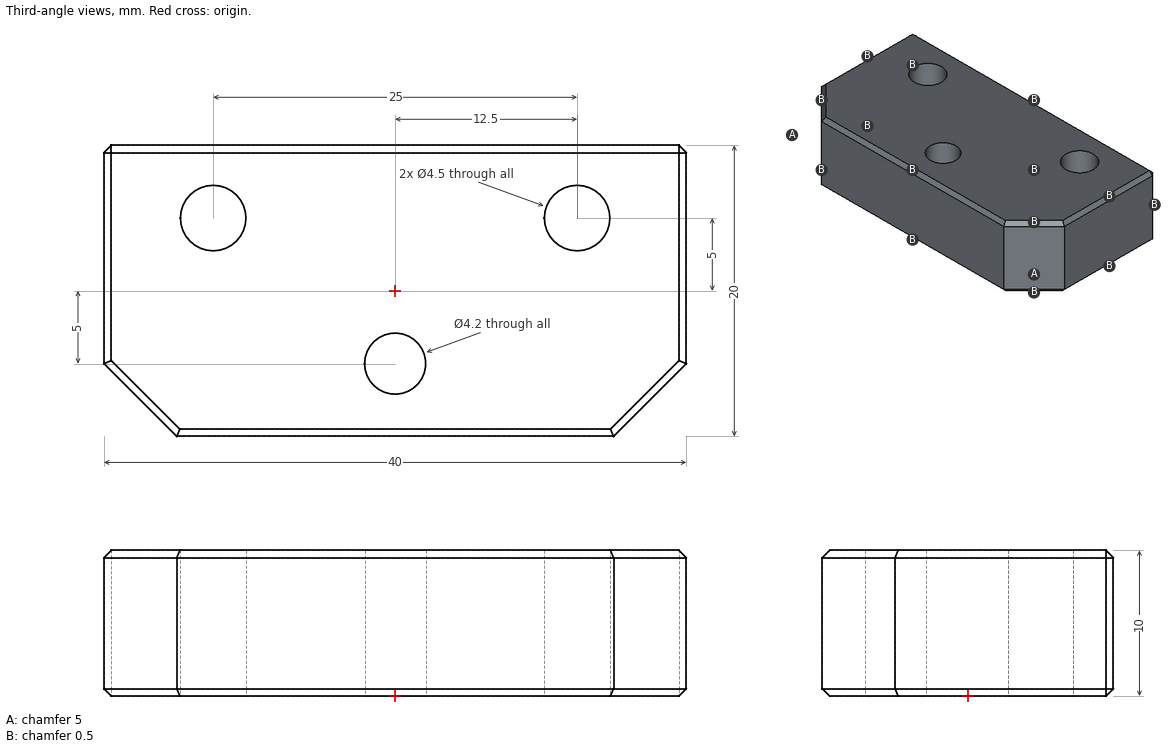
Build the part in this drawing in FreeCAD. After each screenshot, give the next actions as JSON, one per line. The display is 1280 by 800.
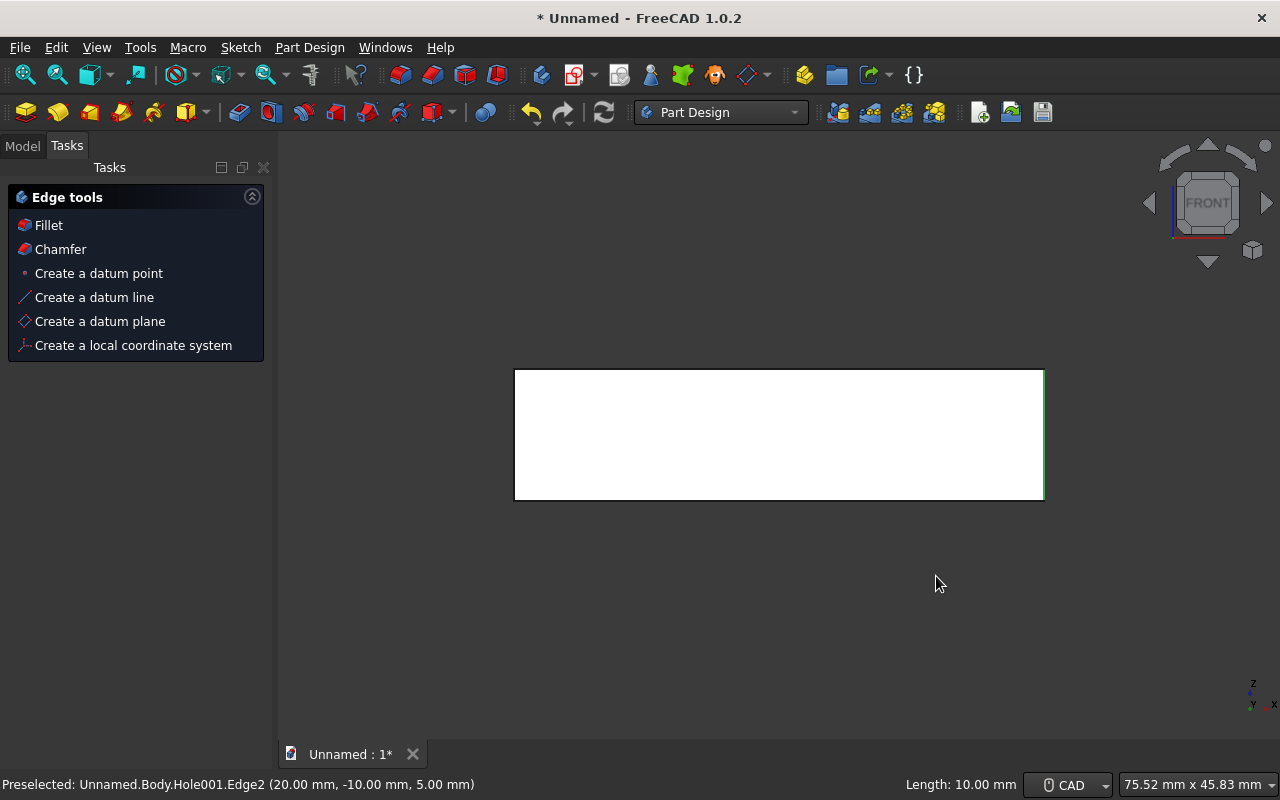
{"action": "left_click", "coordinate": [514, 434], "text": "ctrl"}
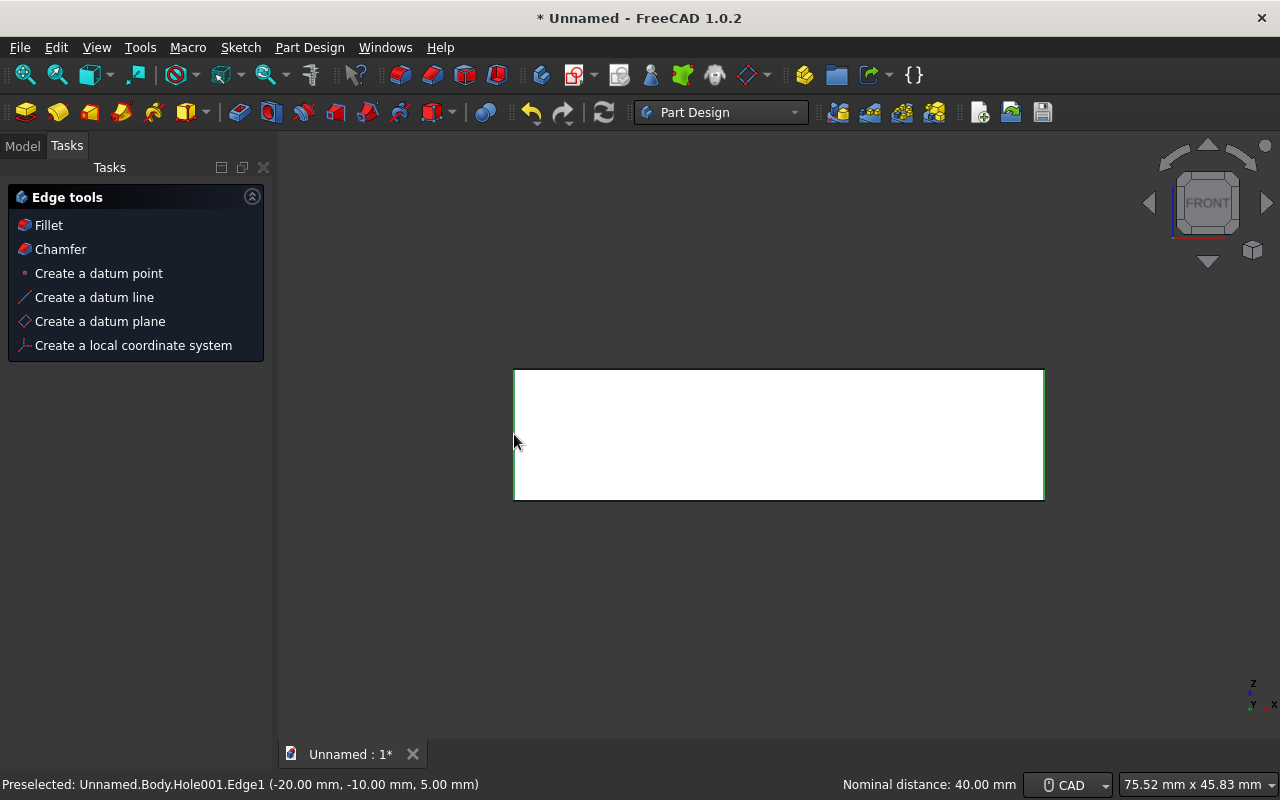
{"action": "left_click", "coordinate": [434, 76]}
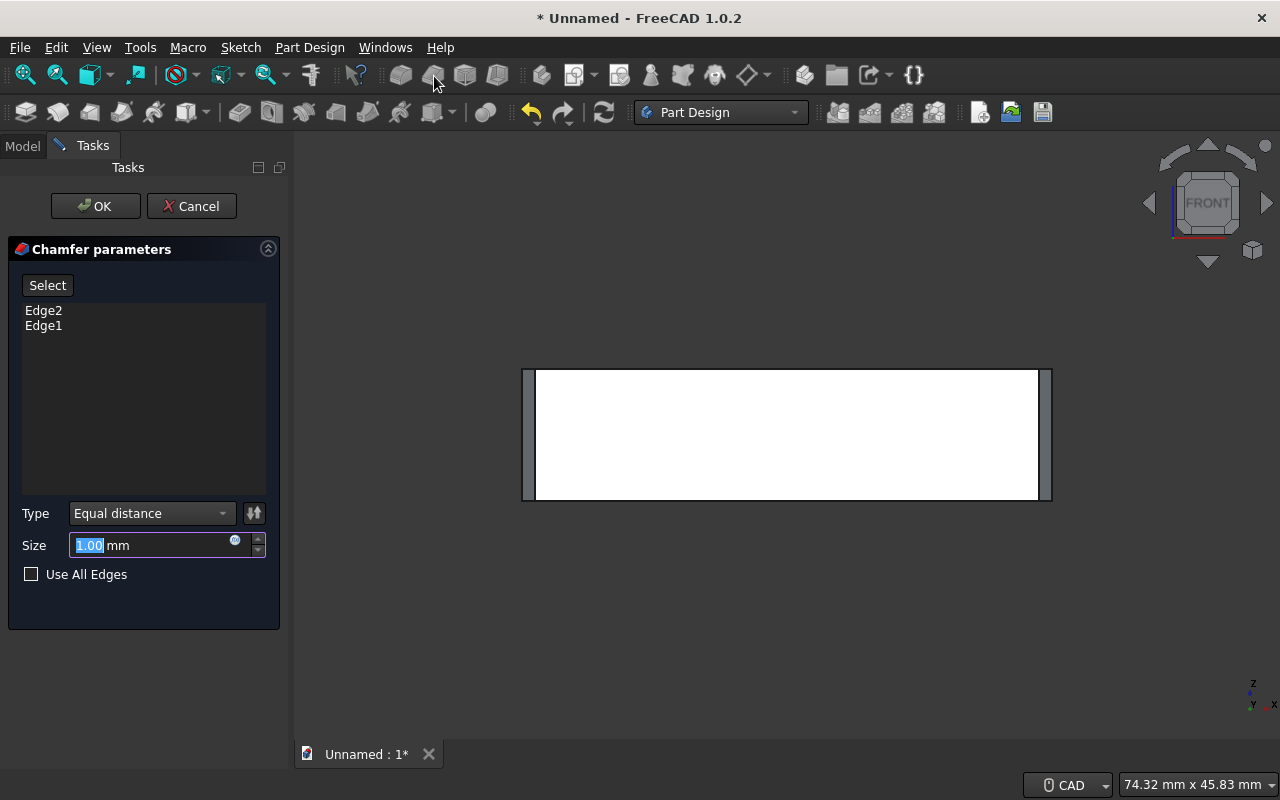
{"action": "type", "text": "5"}
{"action": "key", "text": "Tab"}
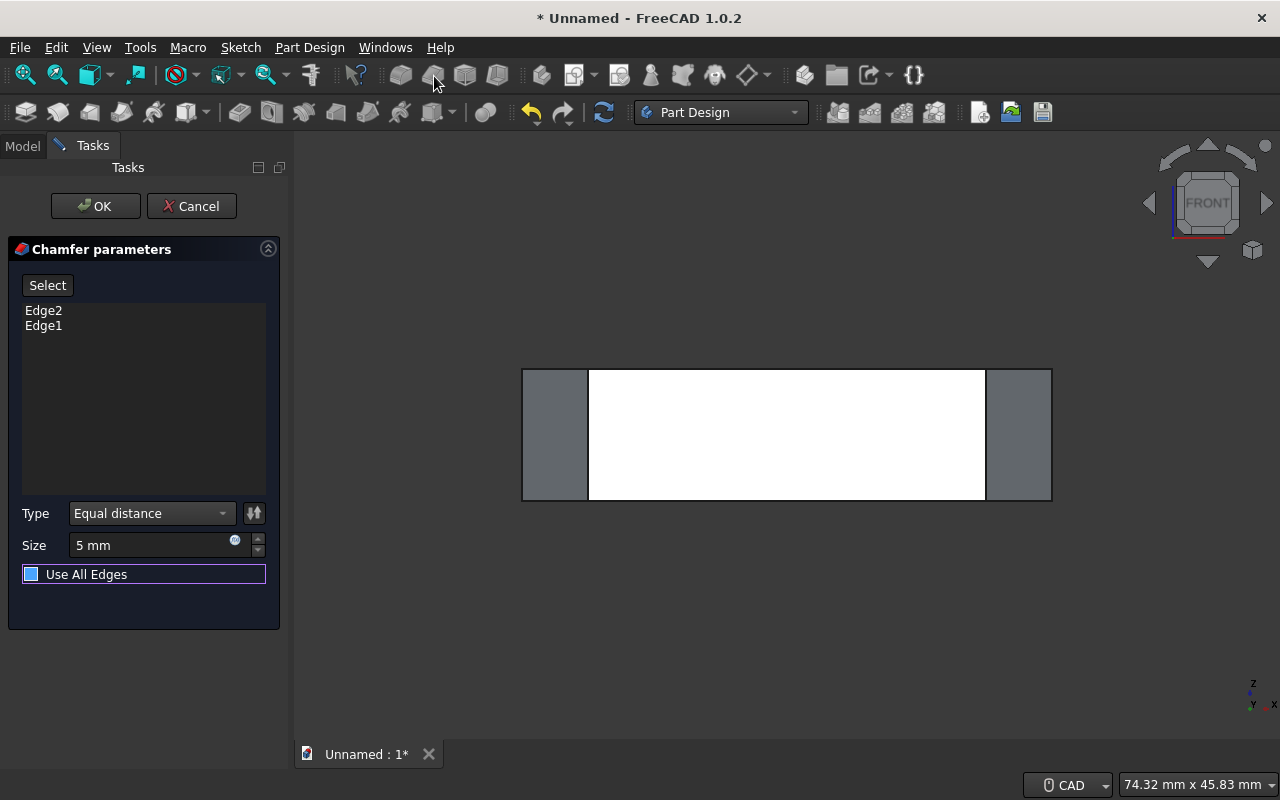
{"action": "left_click", "coordinate": [96, 206]}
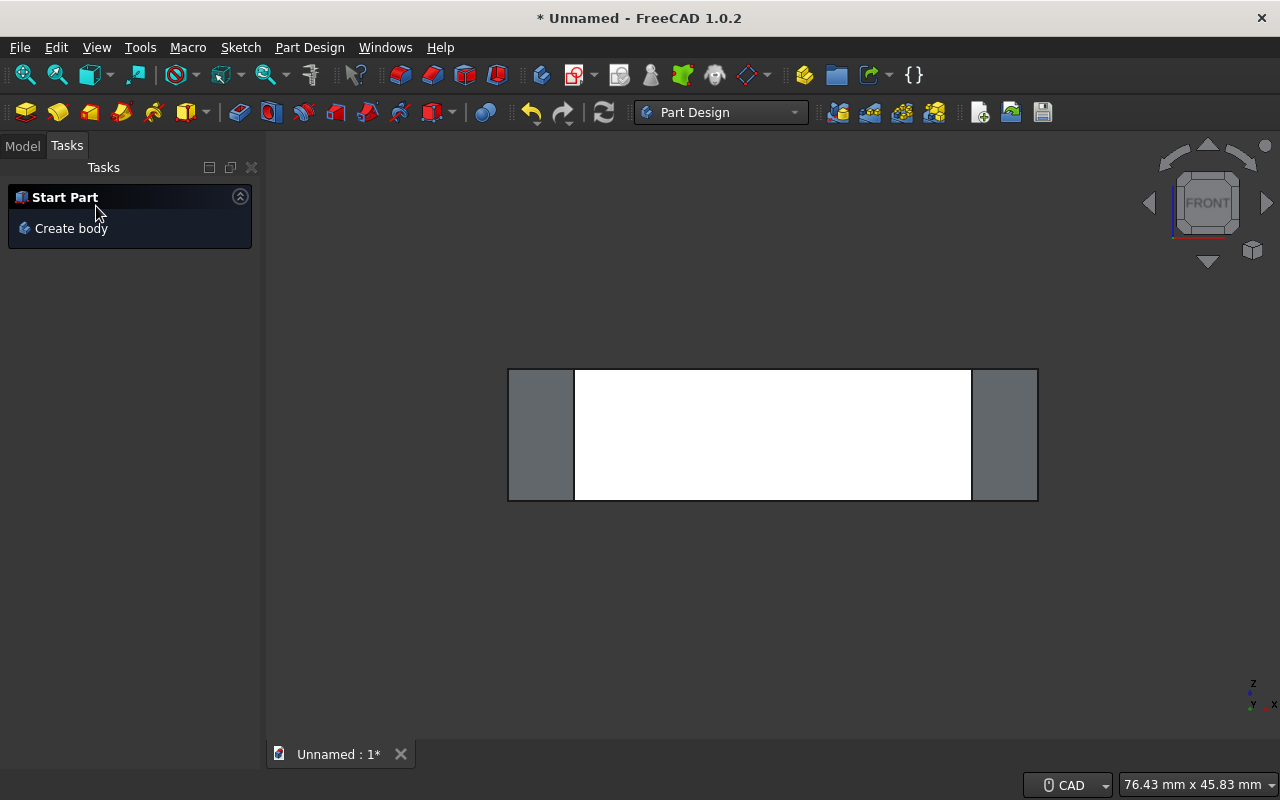
{"action": "left_click", "coordinate": [773, 500]}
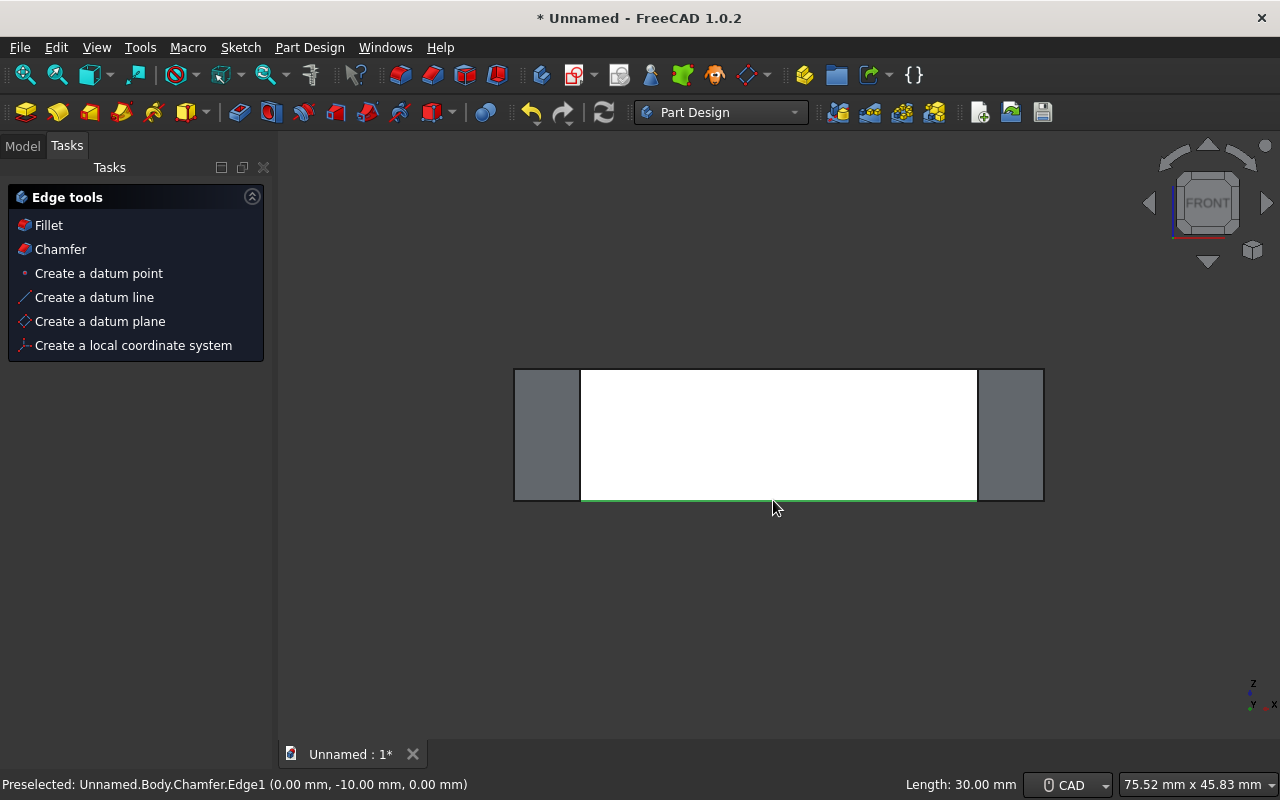
{"action": "left_click", "coordinate": [779, 368], "text": "ctrl"}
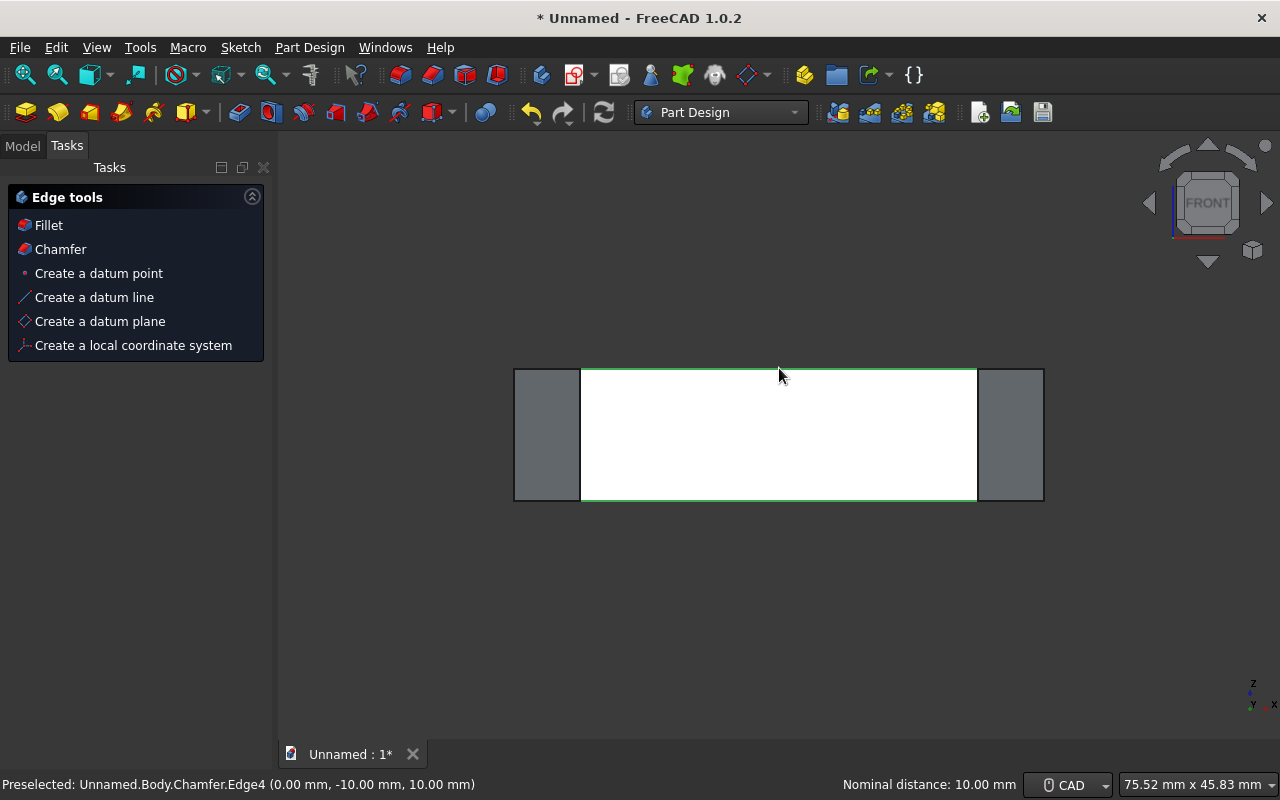
{"action": "left_click", "coordinate": [1011, 500], "text": "ctrl"}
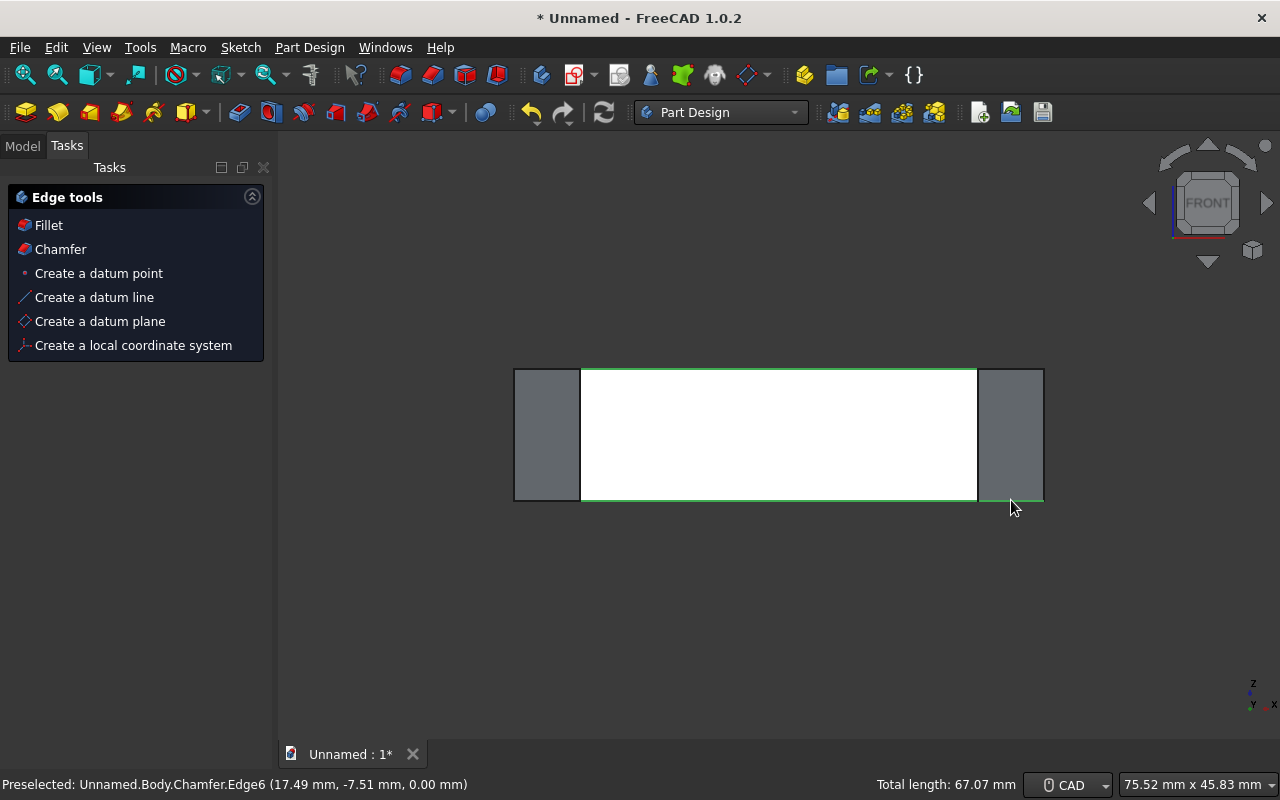
{"action": "left_click", "coordinate": [547, 500], "text": "ctrl"}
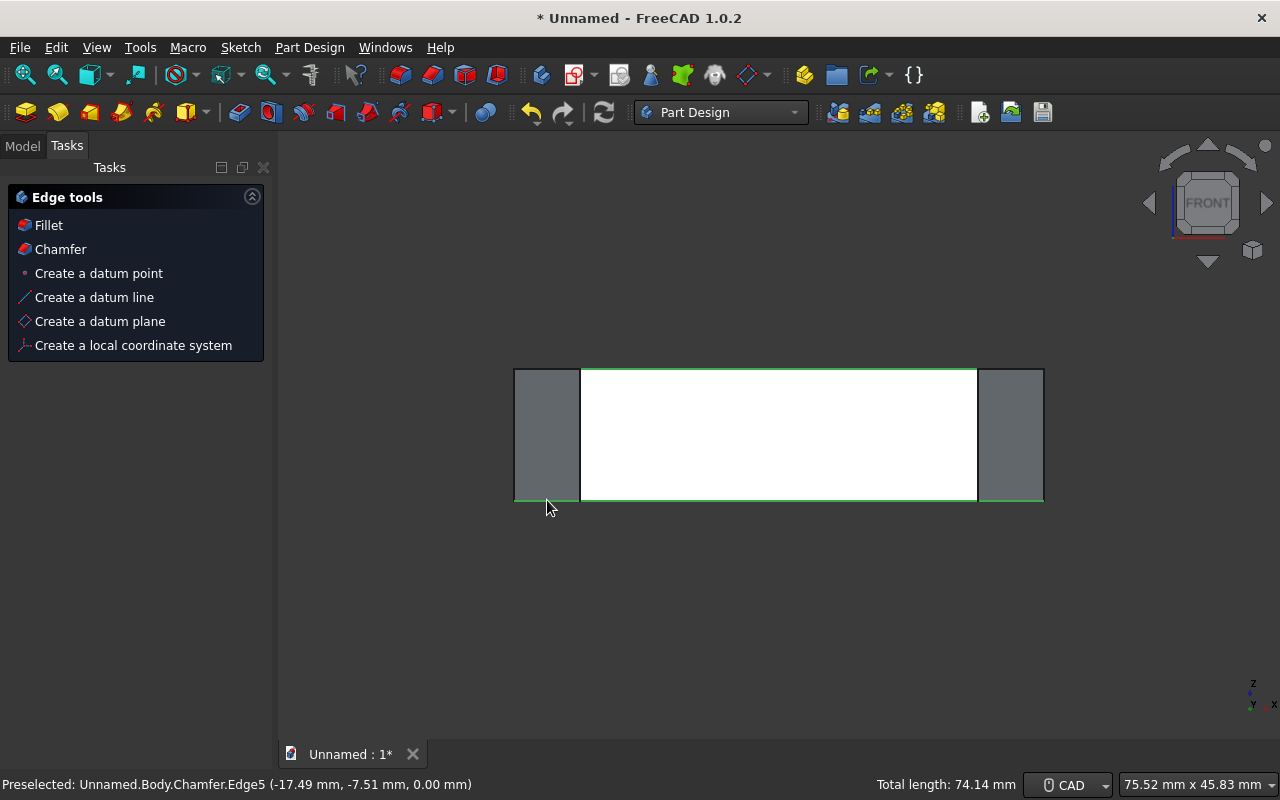
{"action": "left_click", "coordinate": [1011, 368], "text": "ctrl"}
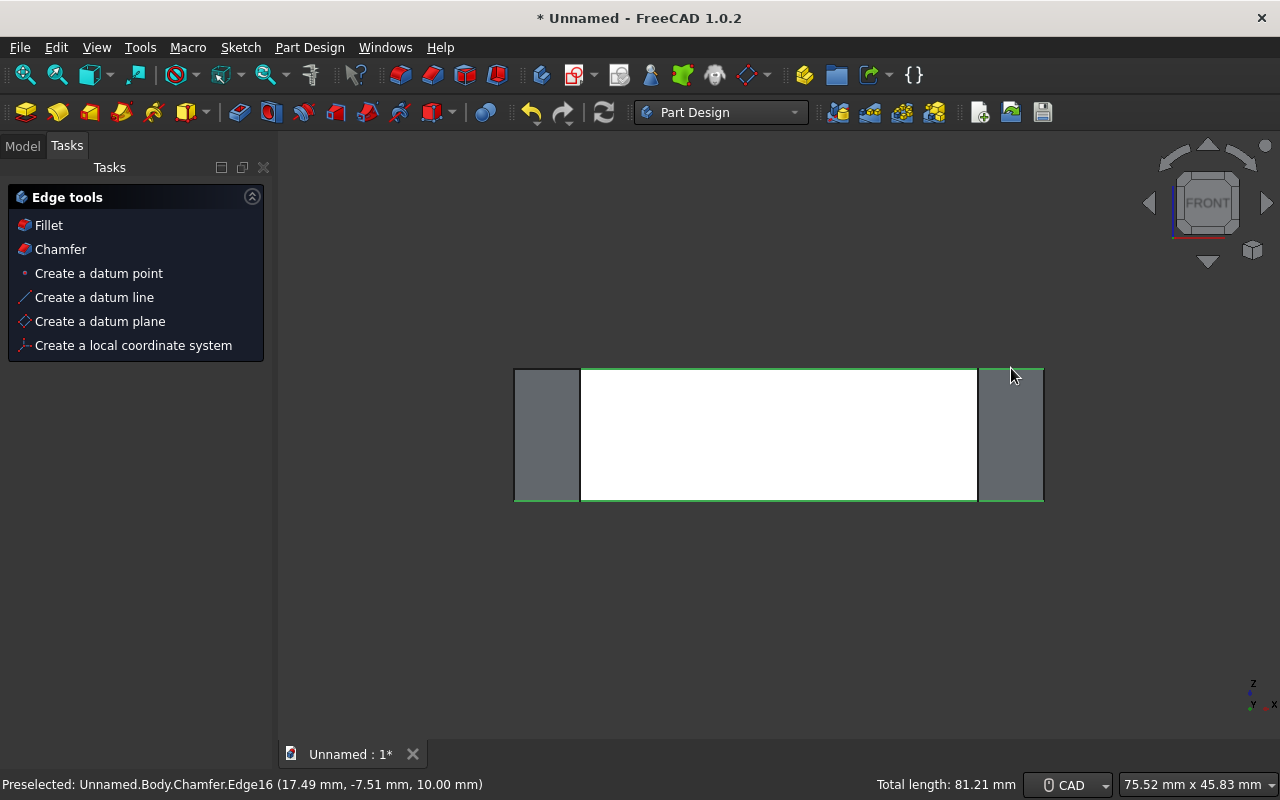
{"action": "left_click", "coordinate": [547, 368], "text": "ctrl"}